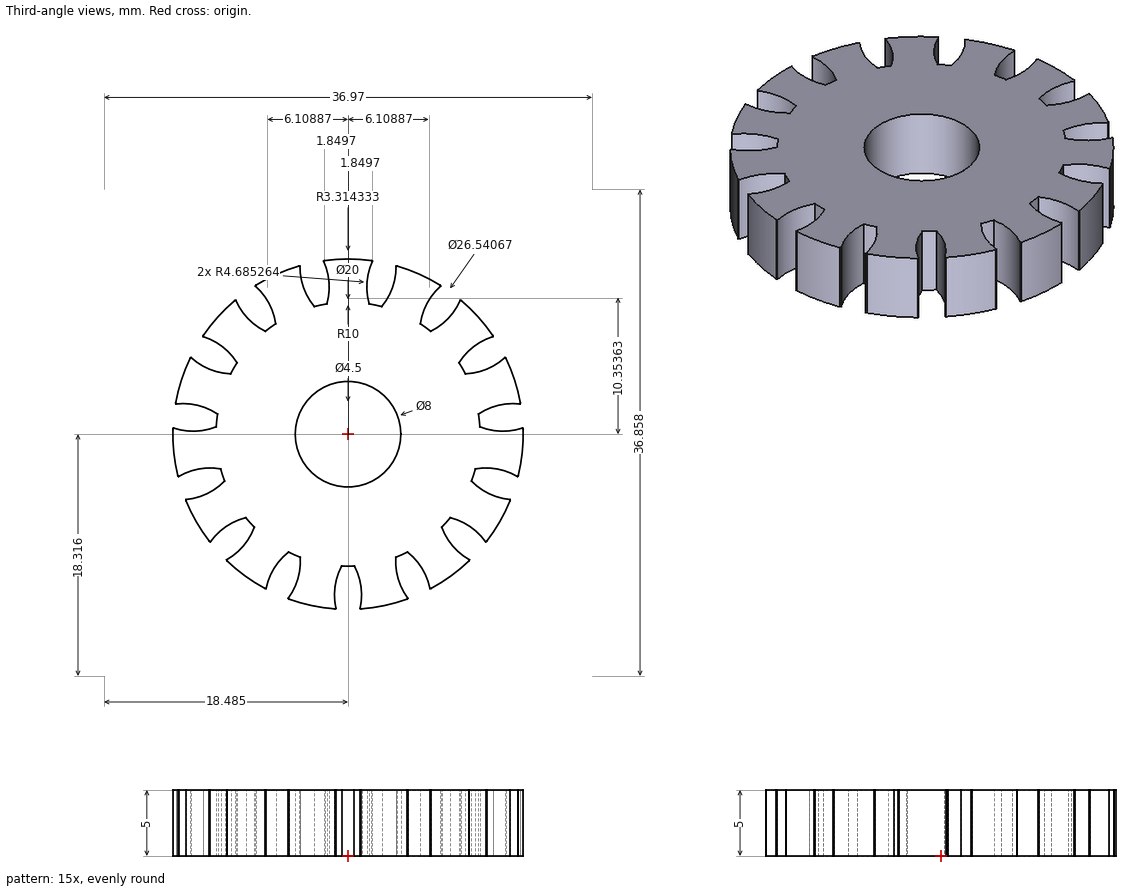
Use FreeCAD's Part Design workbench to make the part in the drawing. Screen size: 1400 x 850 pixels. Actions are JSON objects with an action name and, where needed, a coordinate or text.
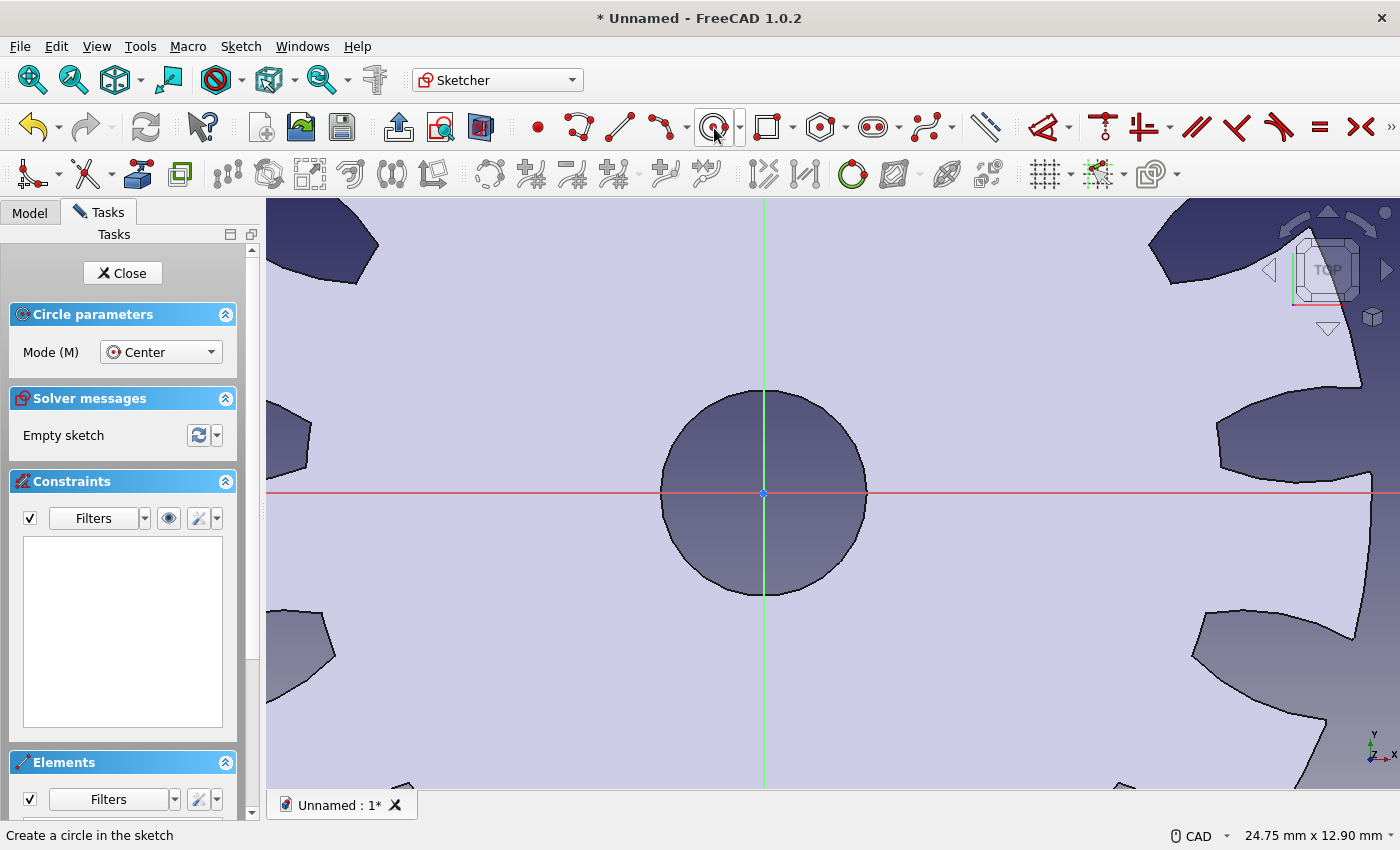
{"action": "left_click", "coordinate": [764, 493]}
{"action": "mouse_move", "coordinate": [893, 363]}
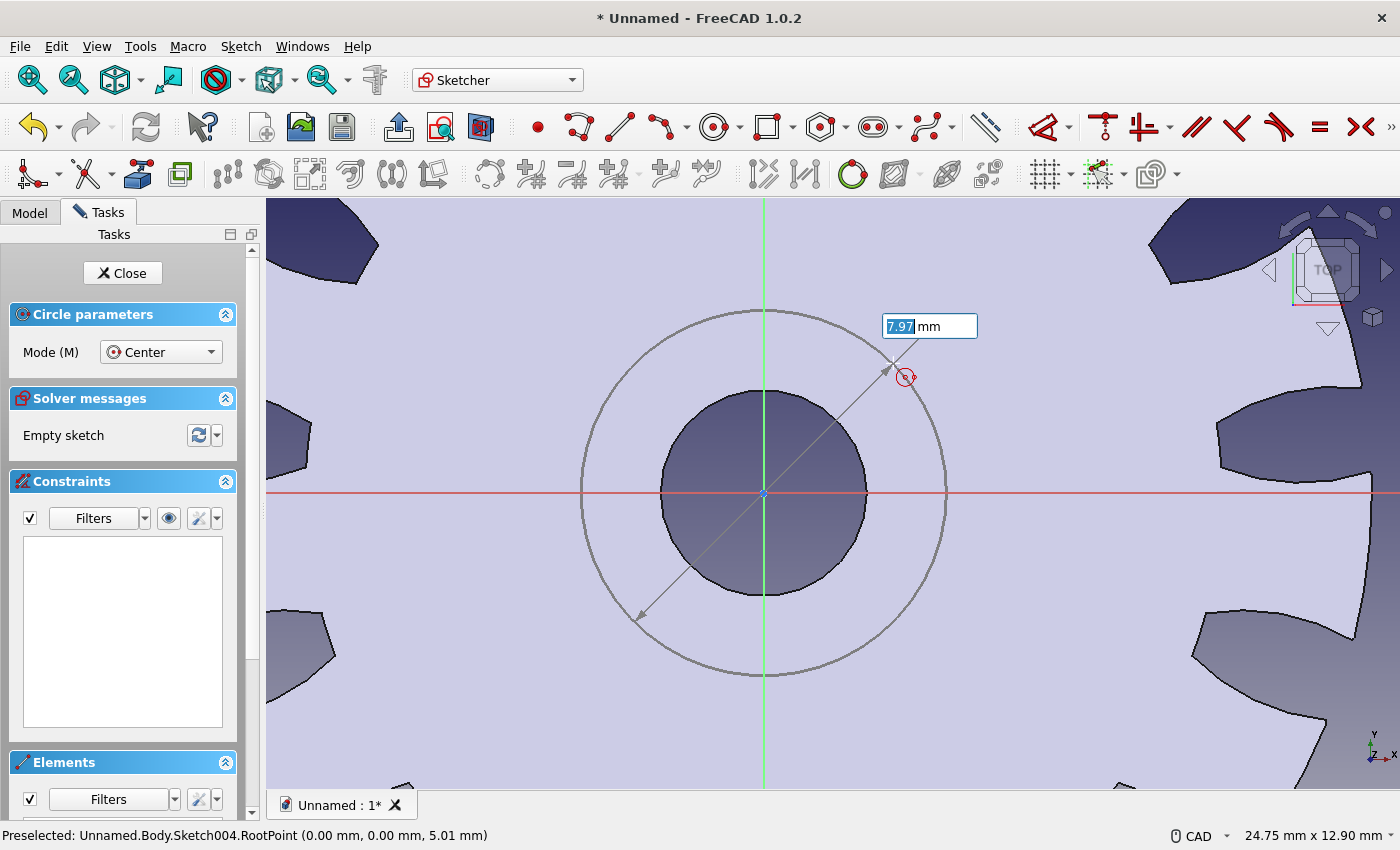
{"action": "type", "text": "8"}
{"action": "key", "text": "Return"}
{"action": "key", "text": "Escape"}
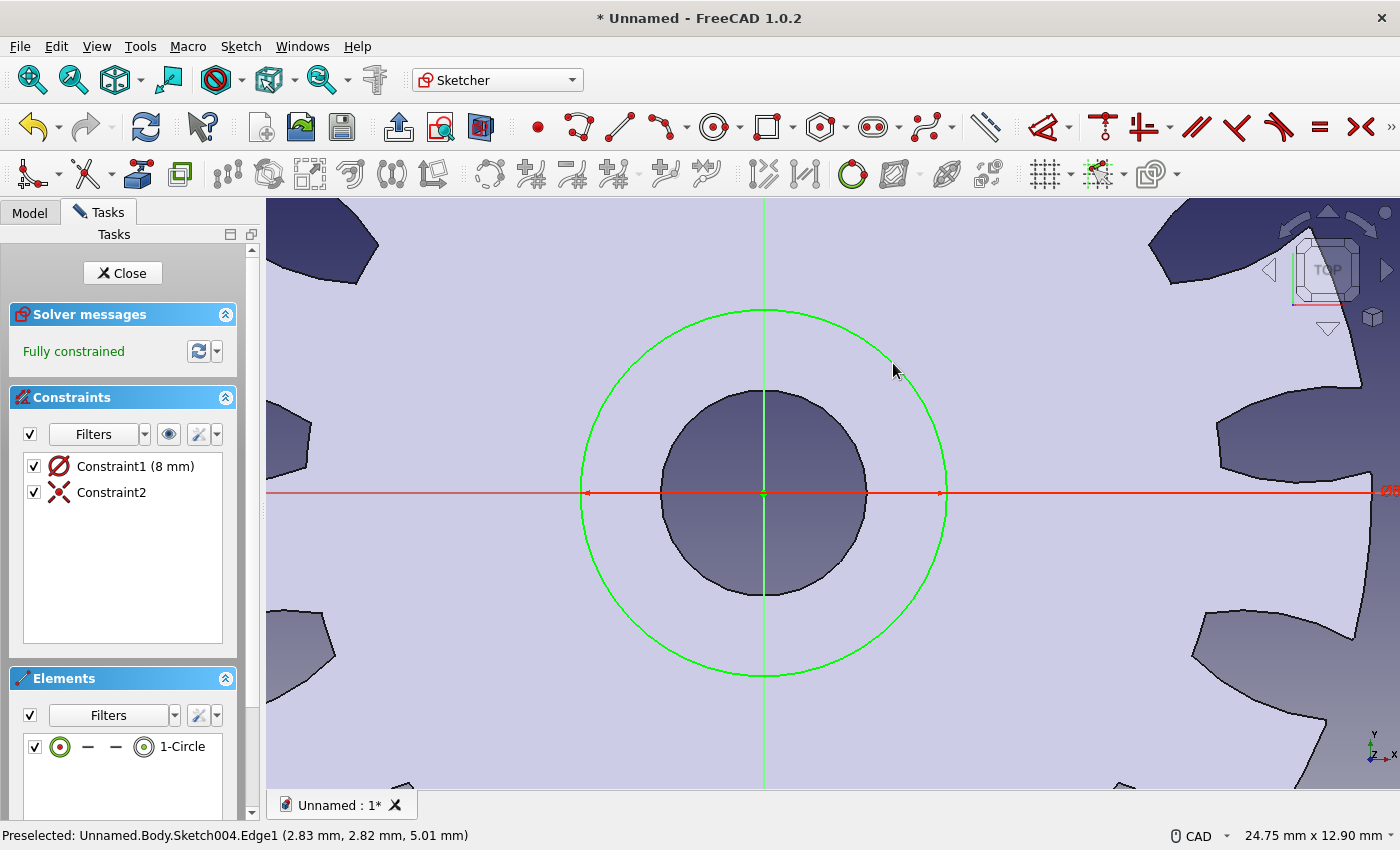
{"action": "left_click", "coordinate": [123, 273]}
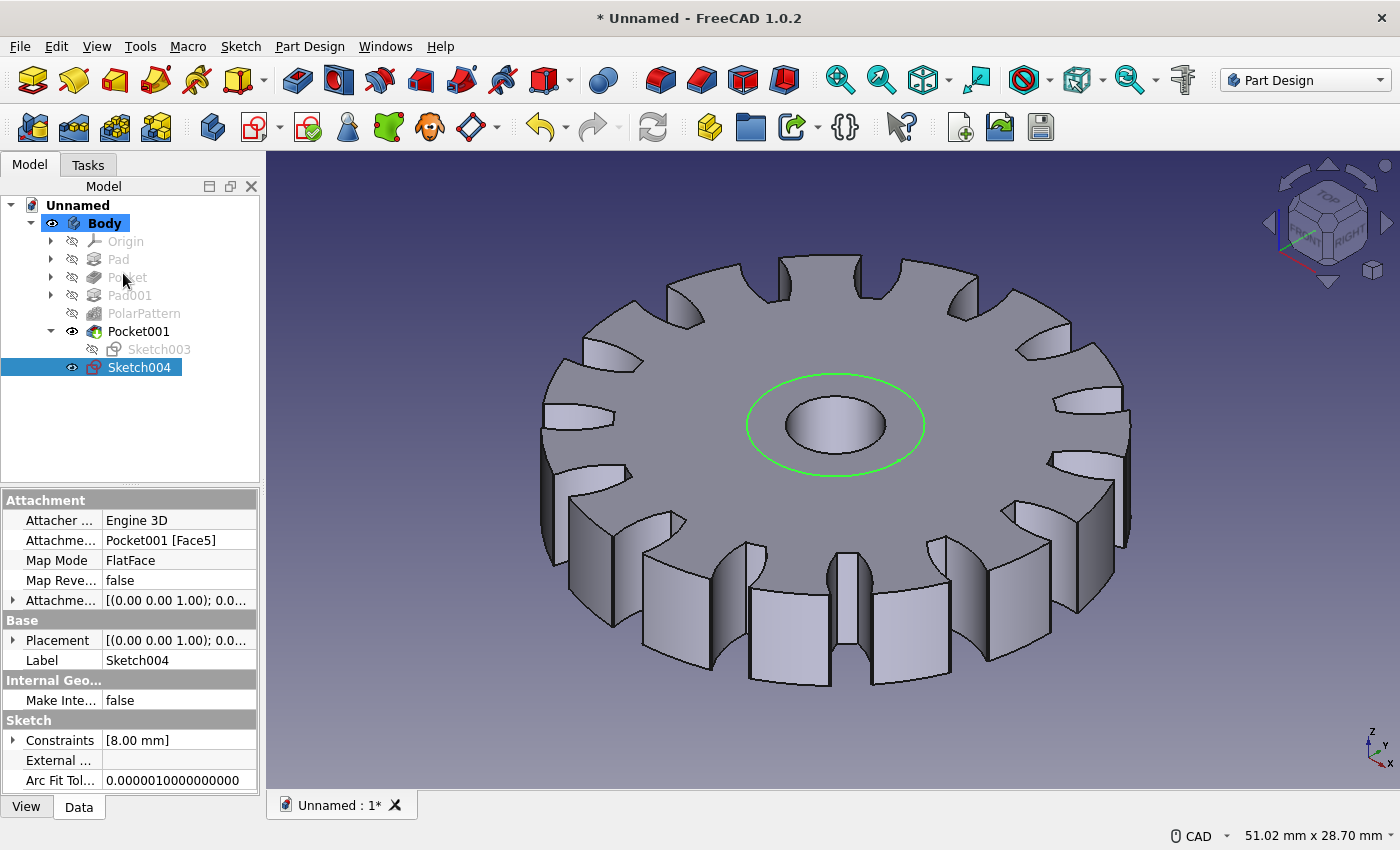
{"action": "left_click", "coordinate": [298, 80]}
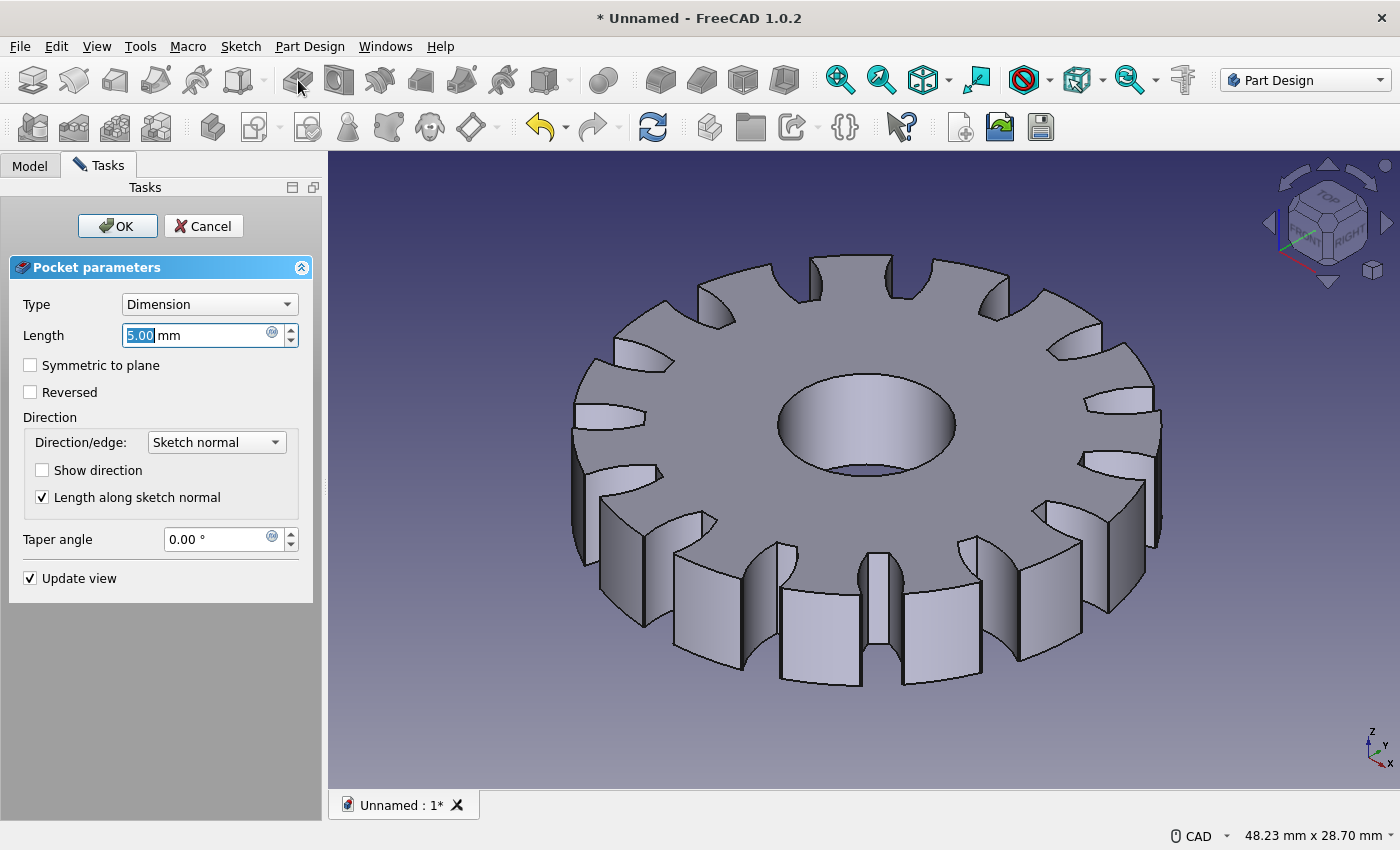
{"action": "left_click", "coordinate": [210, 304]}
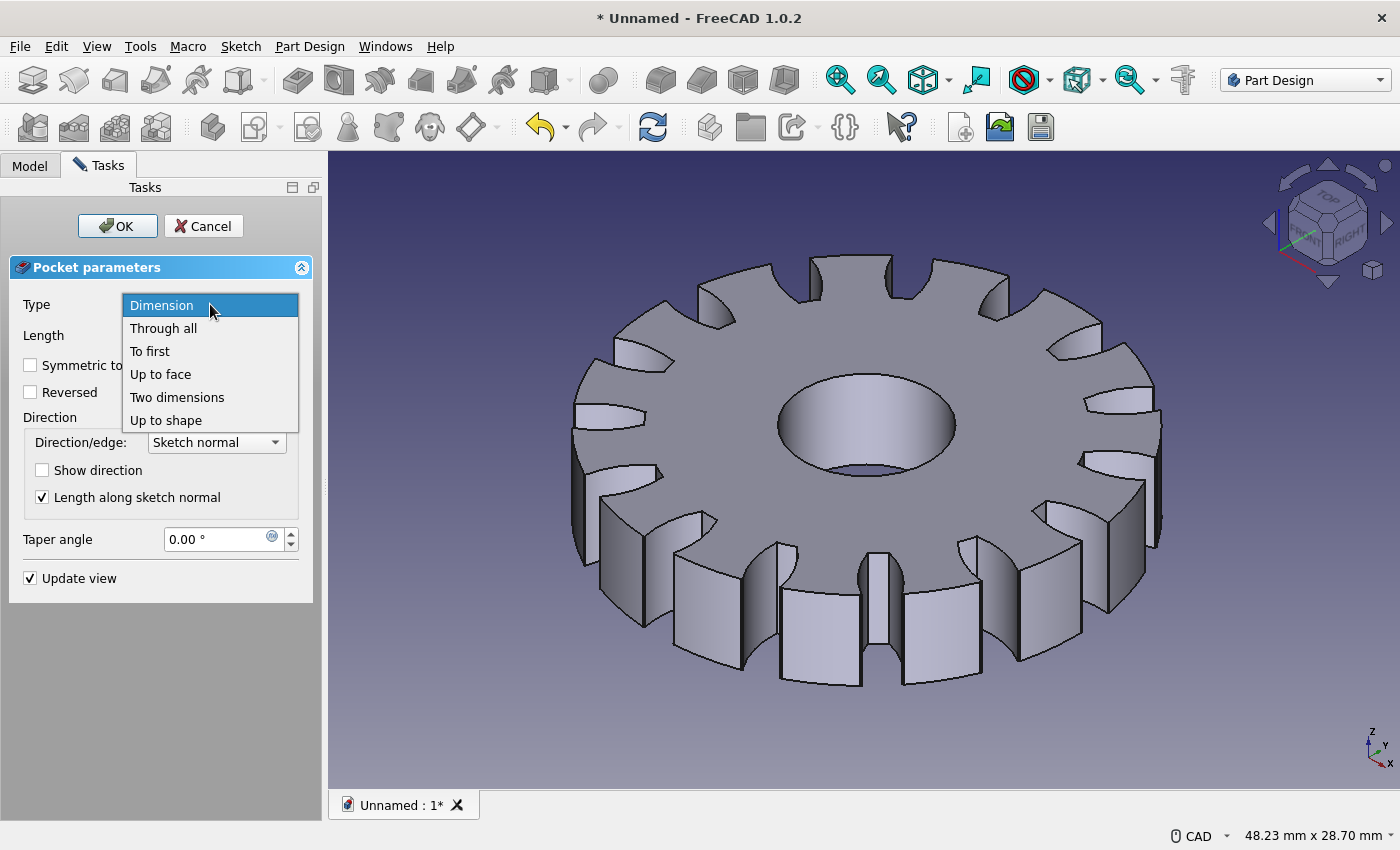
{"action": "left_click", "coordinate": [208, 328]}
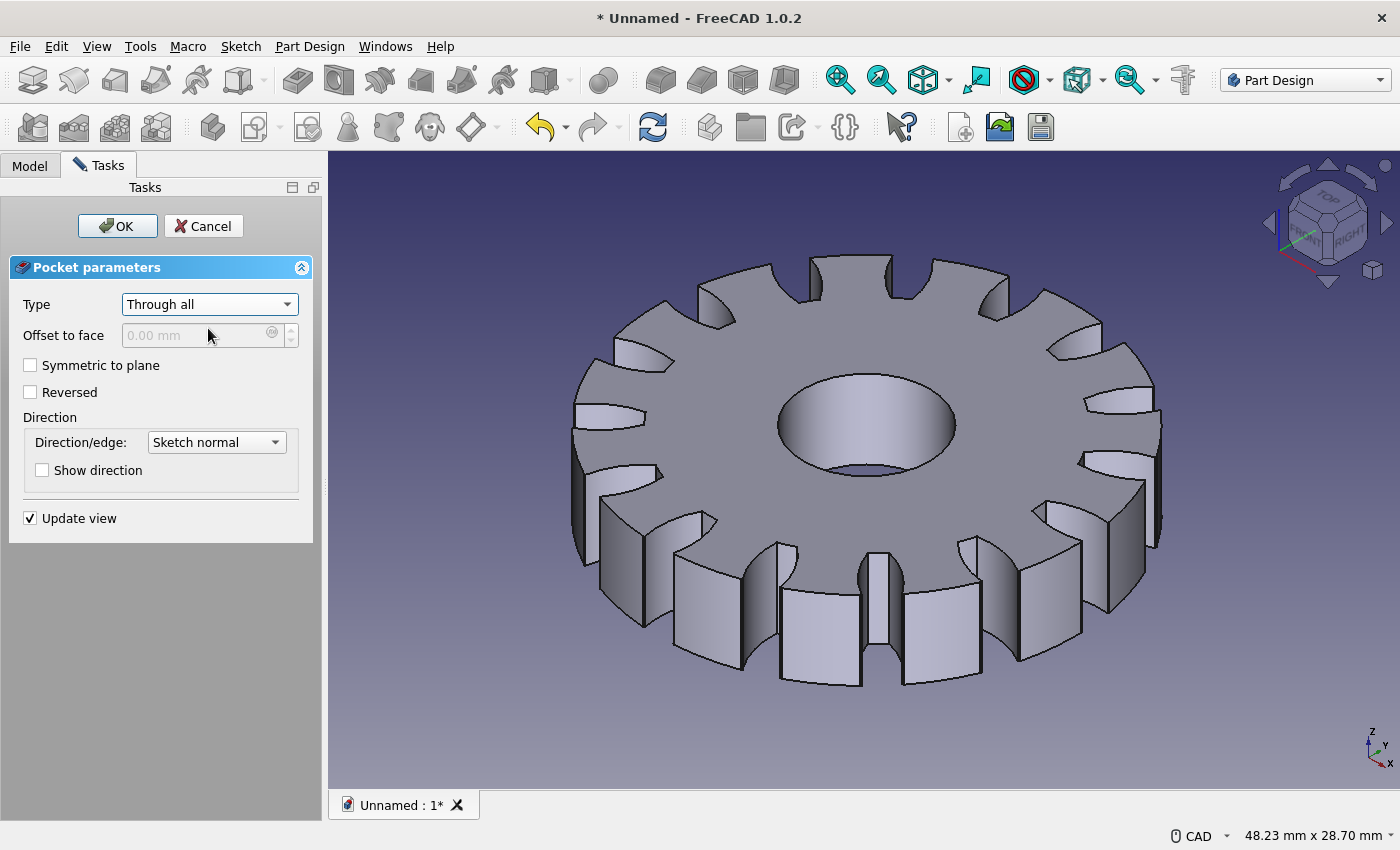
{"action": "left_click", "coordinate": [118, 226]}